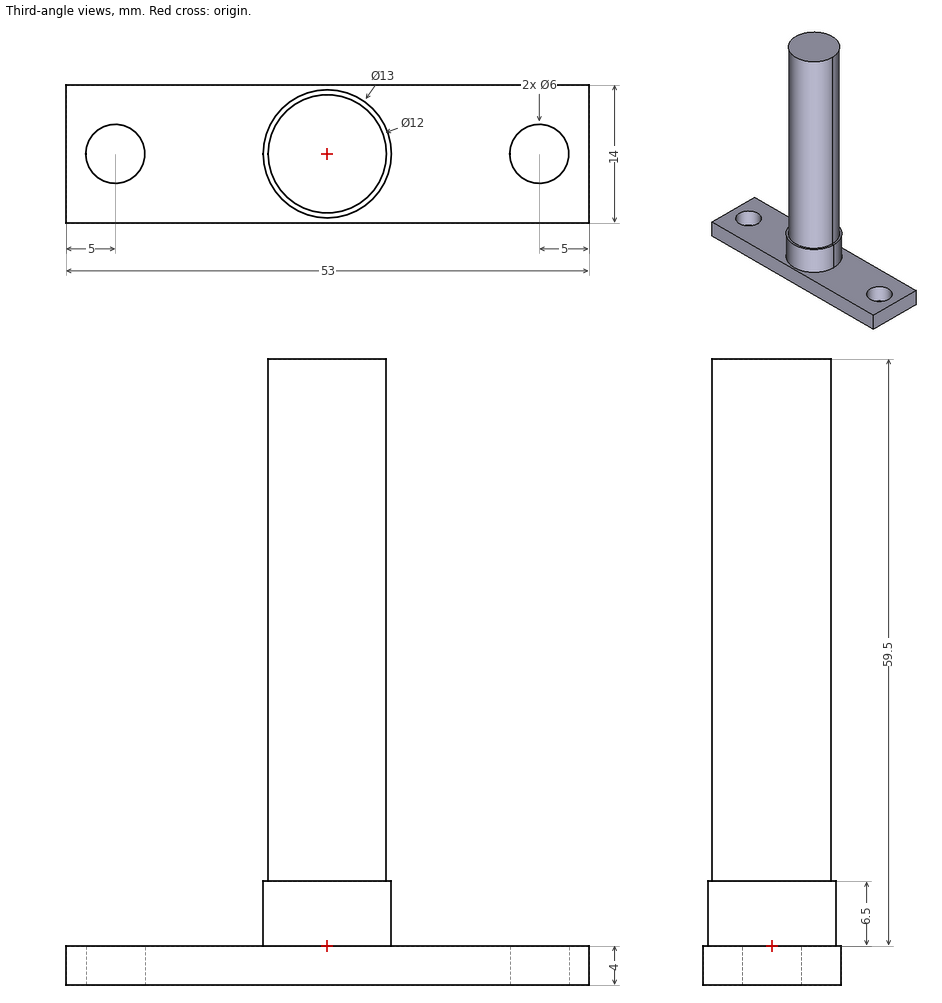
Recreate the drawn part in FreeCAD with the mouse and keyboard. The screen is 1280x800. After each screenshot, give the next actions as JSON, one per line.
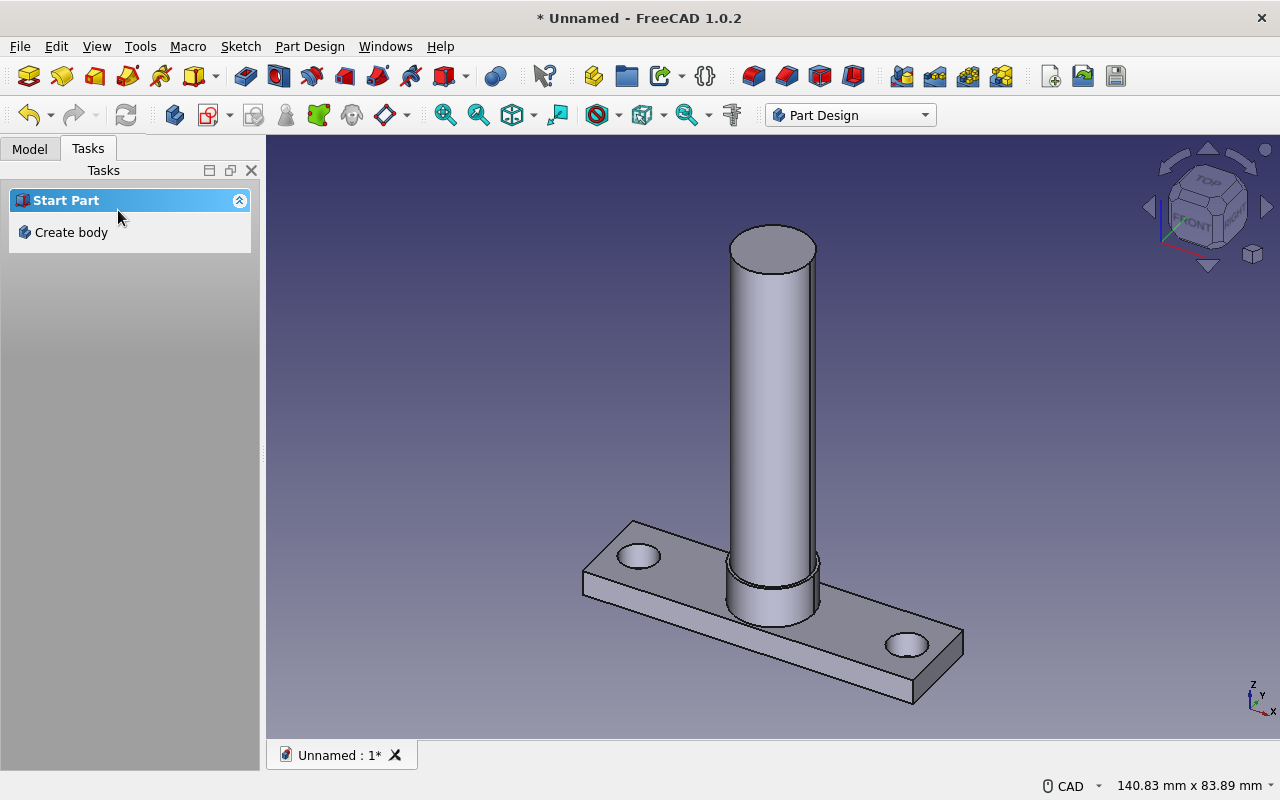
{"action": "key", "text": "0"}